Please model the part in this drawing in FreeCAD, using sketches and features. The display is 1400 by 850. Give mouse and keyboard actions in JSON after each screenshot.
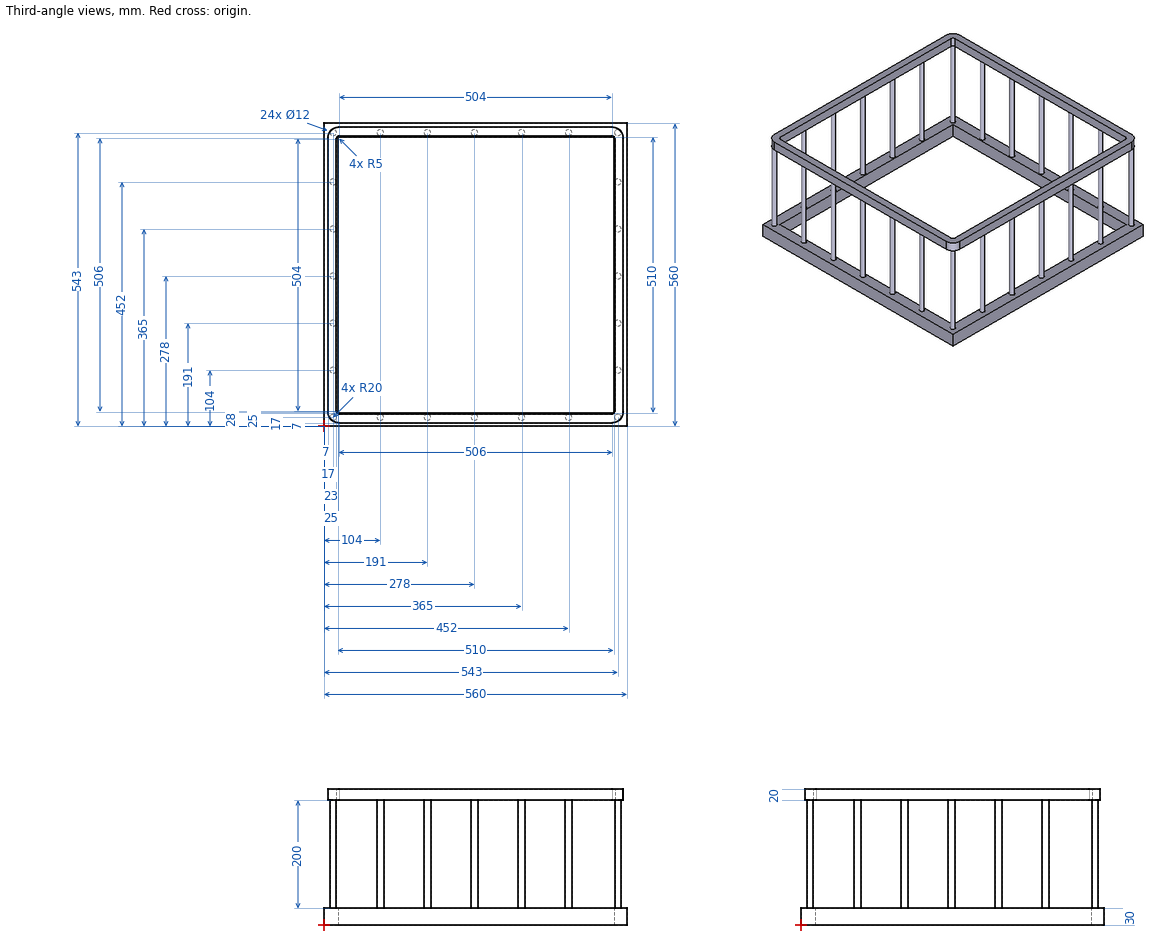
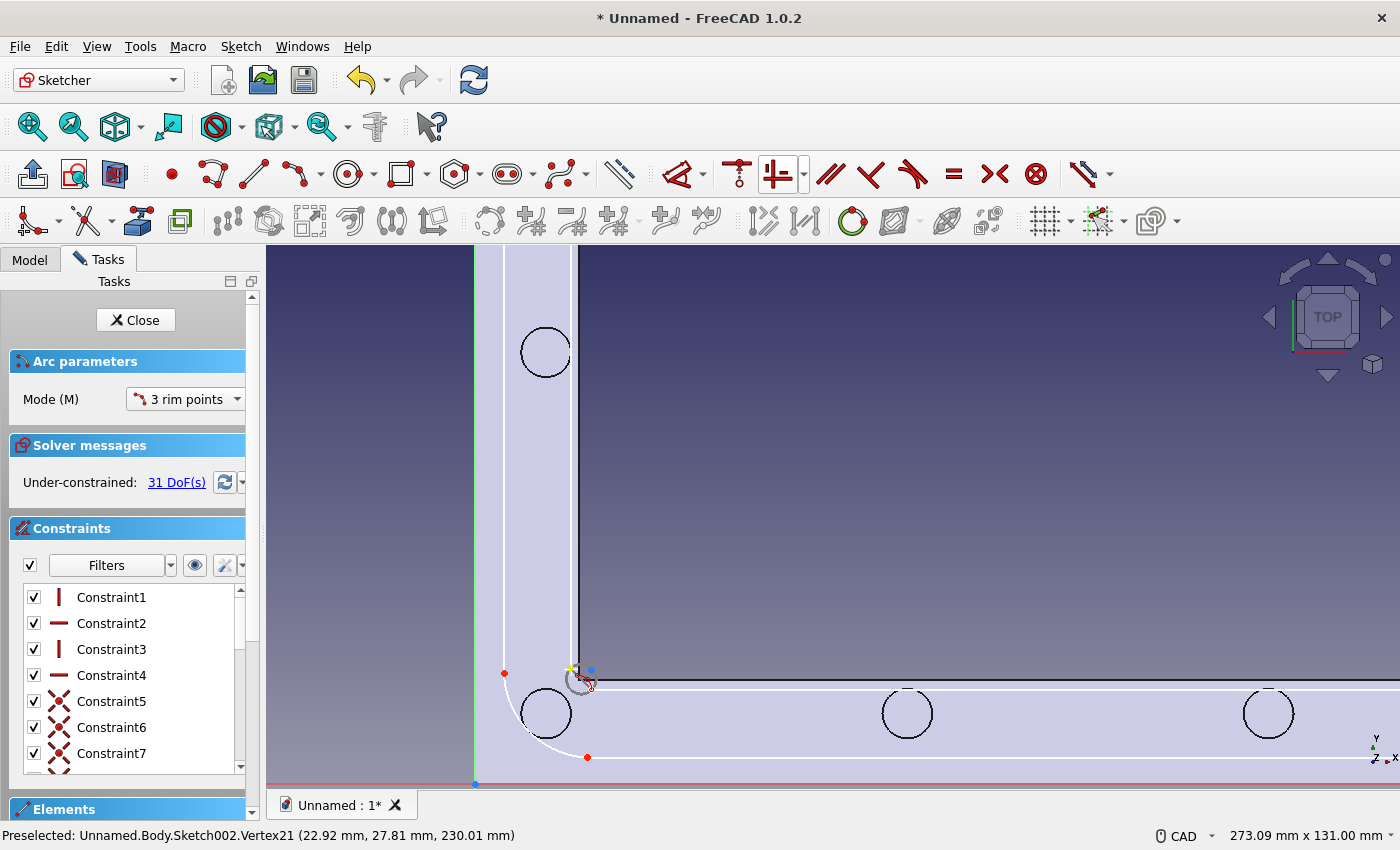
{"action": "scroll", "coordinate": [577, 683], "scroll_direction": "up", "scroll_amount": 5}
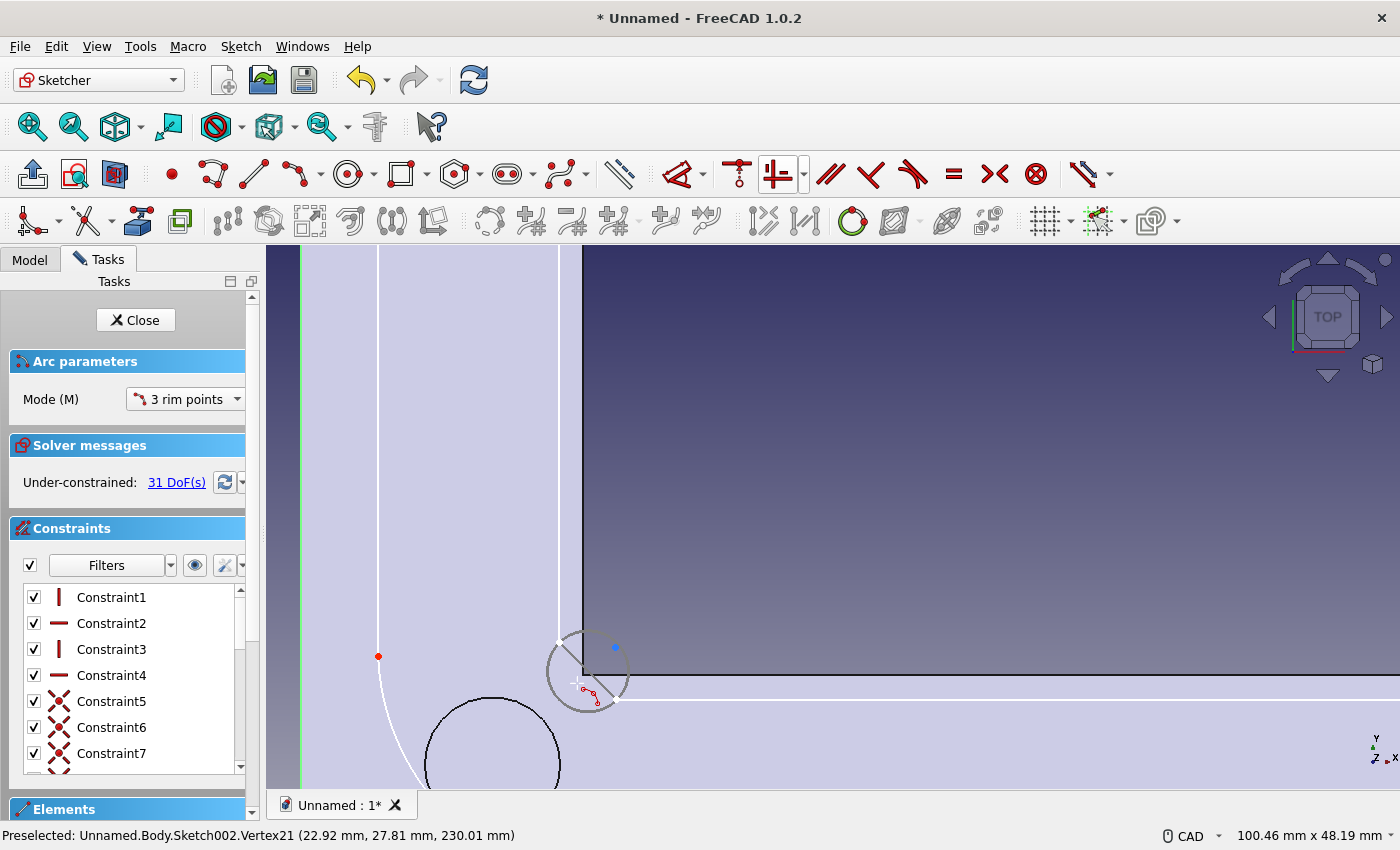
{"action": "left_click", "coordinate": [577, 681]}
{"action": "key", "text": "Escape"}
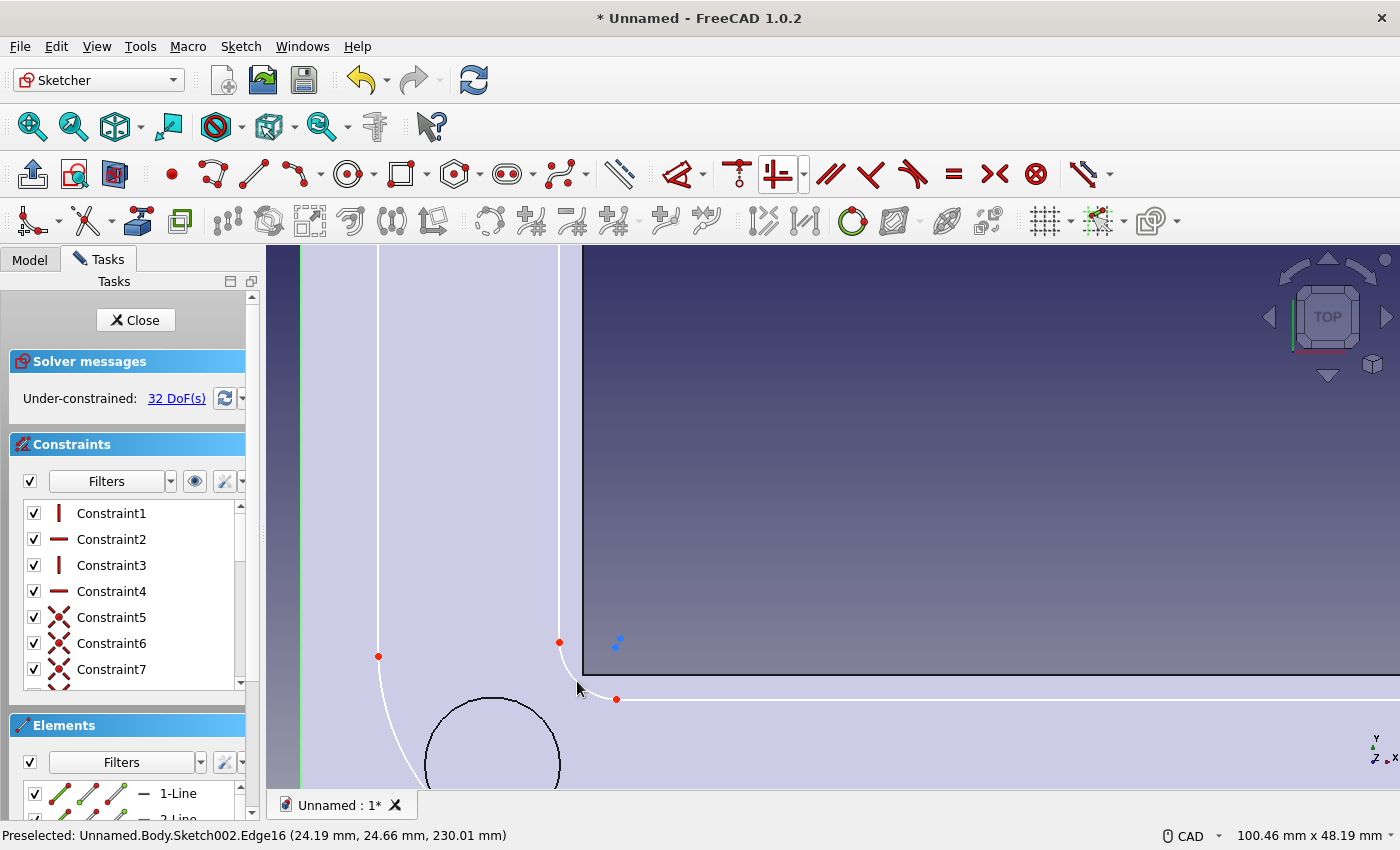
{"action": "scroll", "coordinate": [592, 691], "scroll_direction": "down", "scroll_amount": 14}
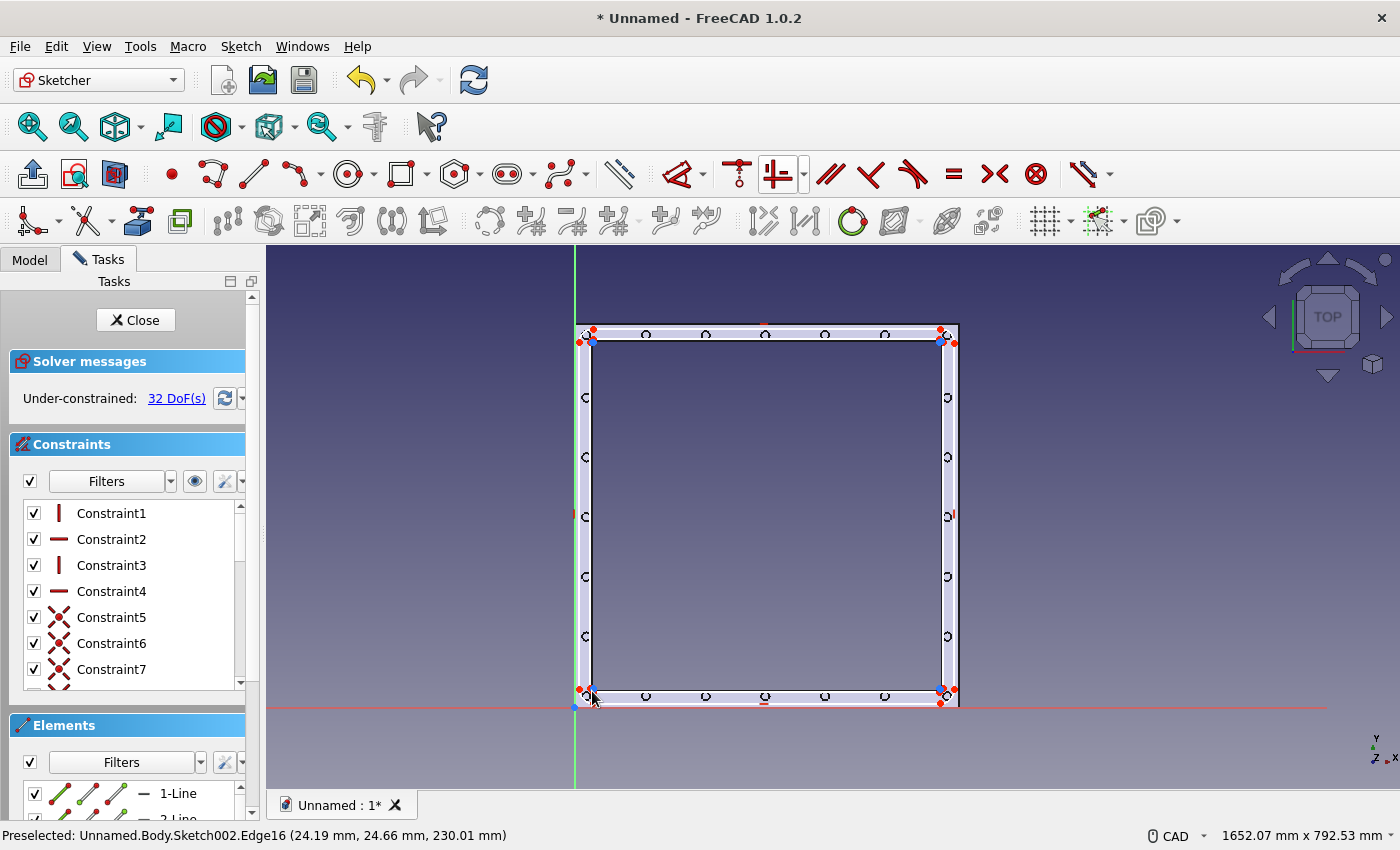
{"action": "scroll", "coordinate": [579, 447], "scroll_direction": "up", "scroll_amount": 6}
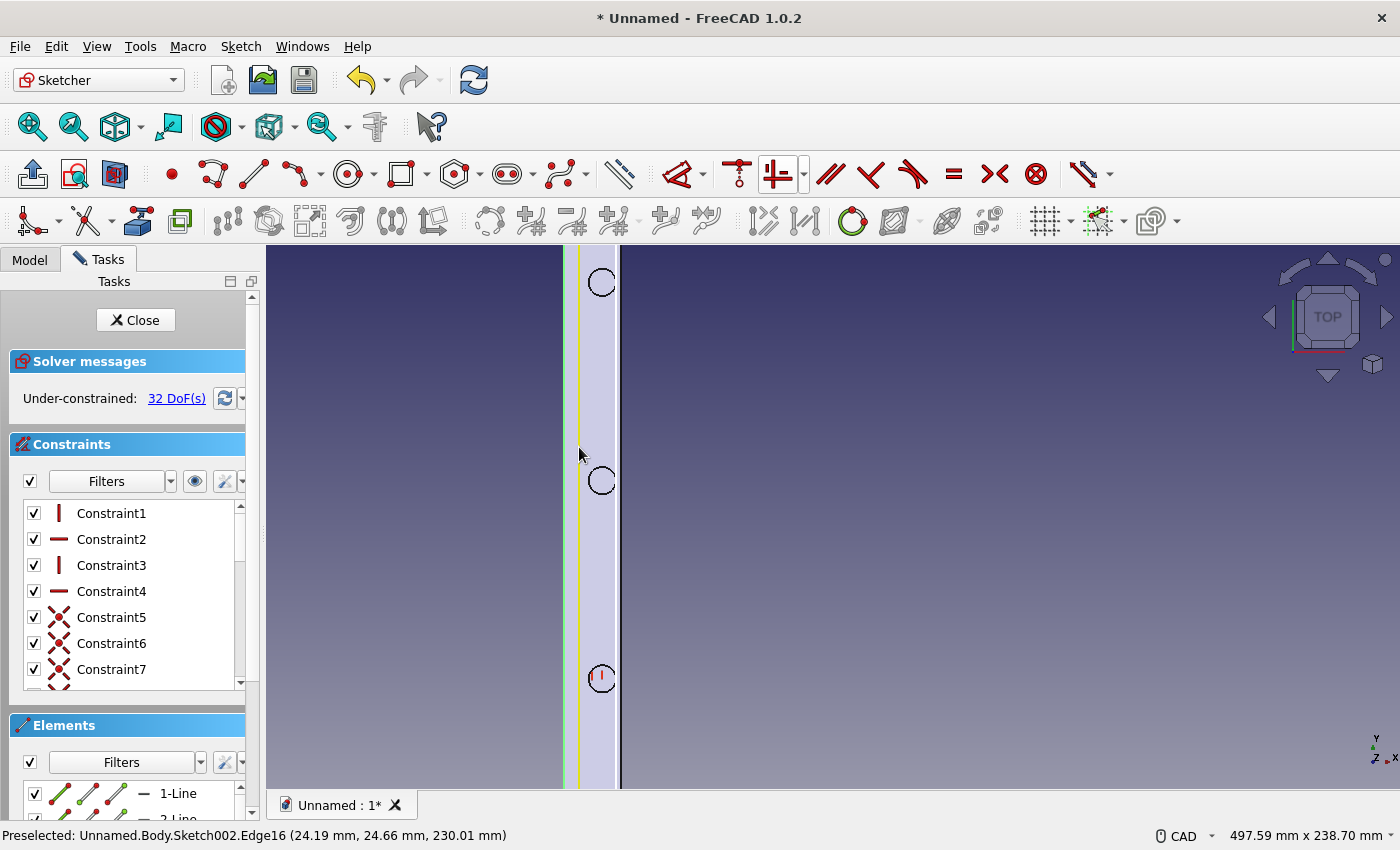
{"action": "left_click", "coordinate": [579, 445]}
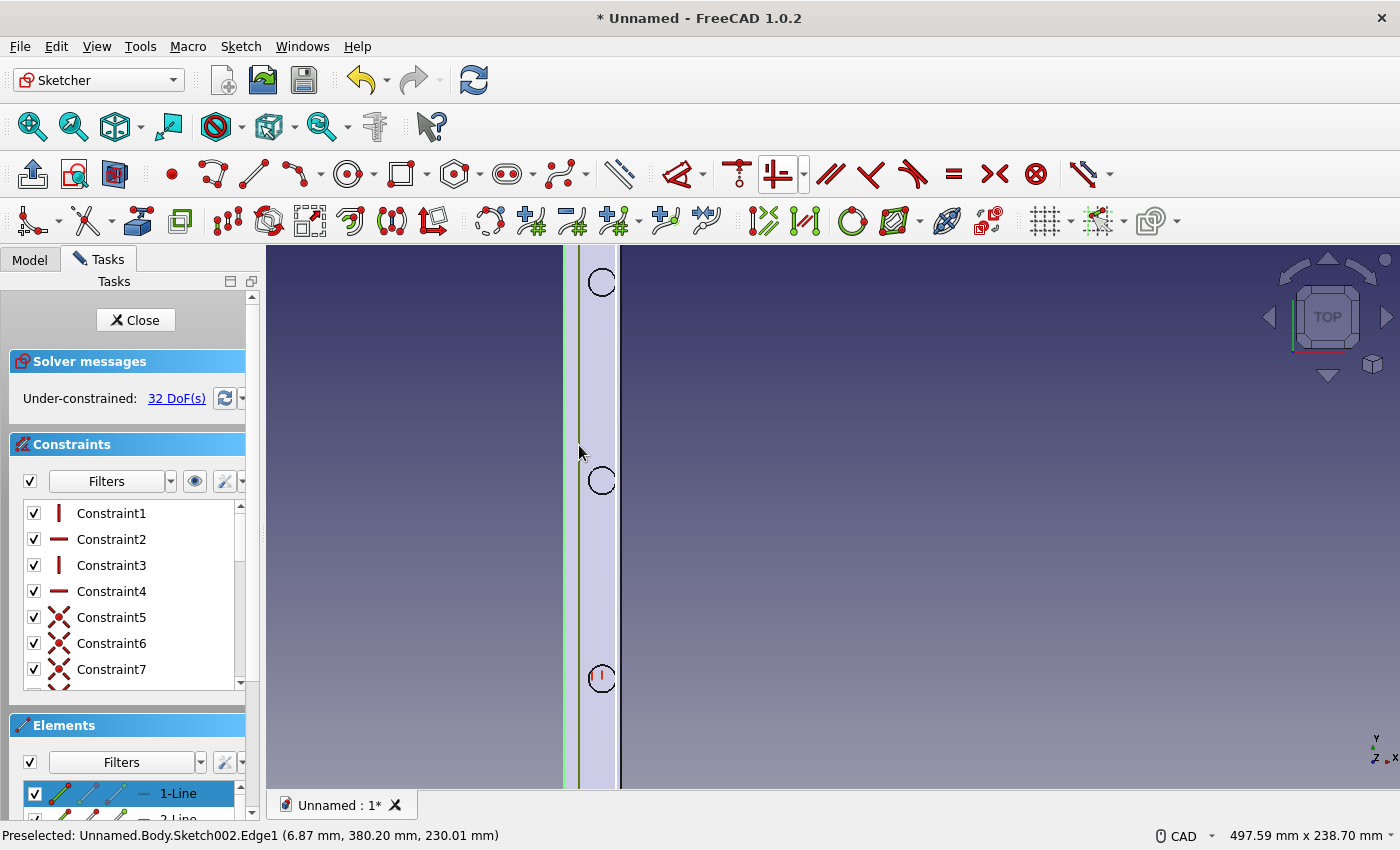
{"action": "scroll", "coordinate": [580, 446], "scroll_direction": "down", "scroll_amount": 6}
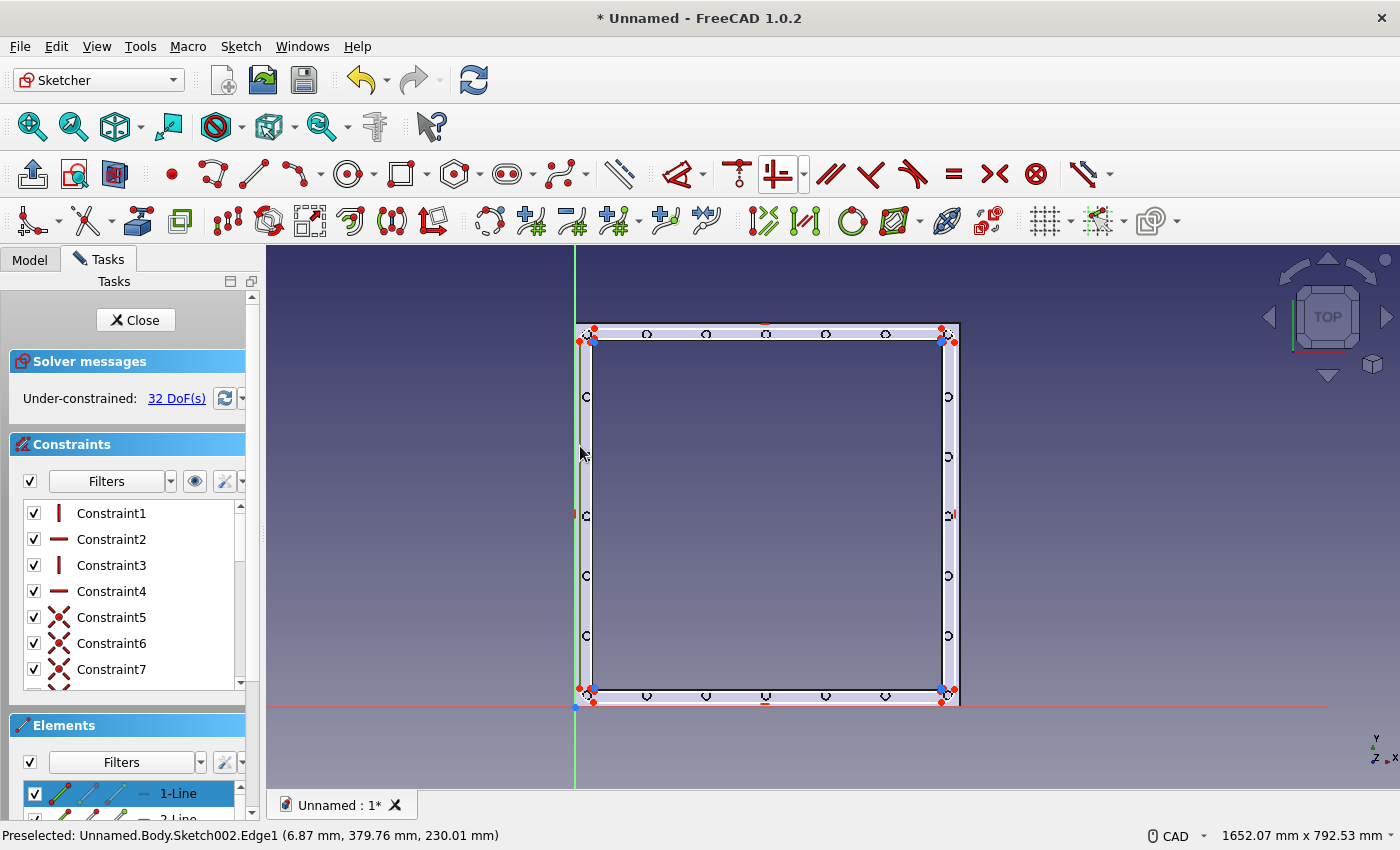
{"action": "scroll", "coordinate": [582, 695], "scroll_direction": "up", "scroll_amount": 4}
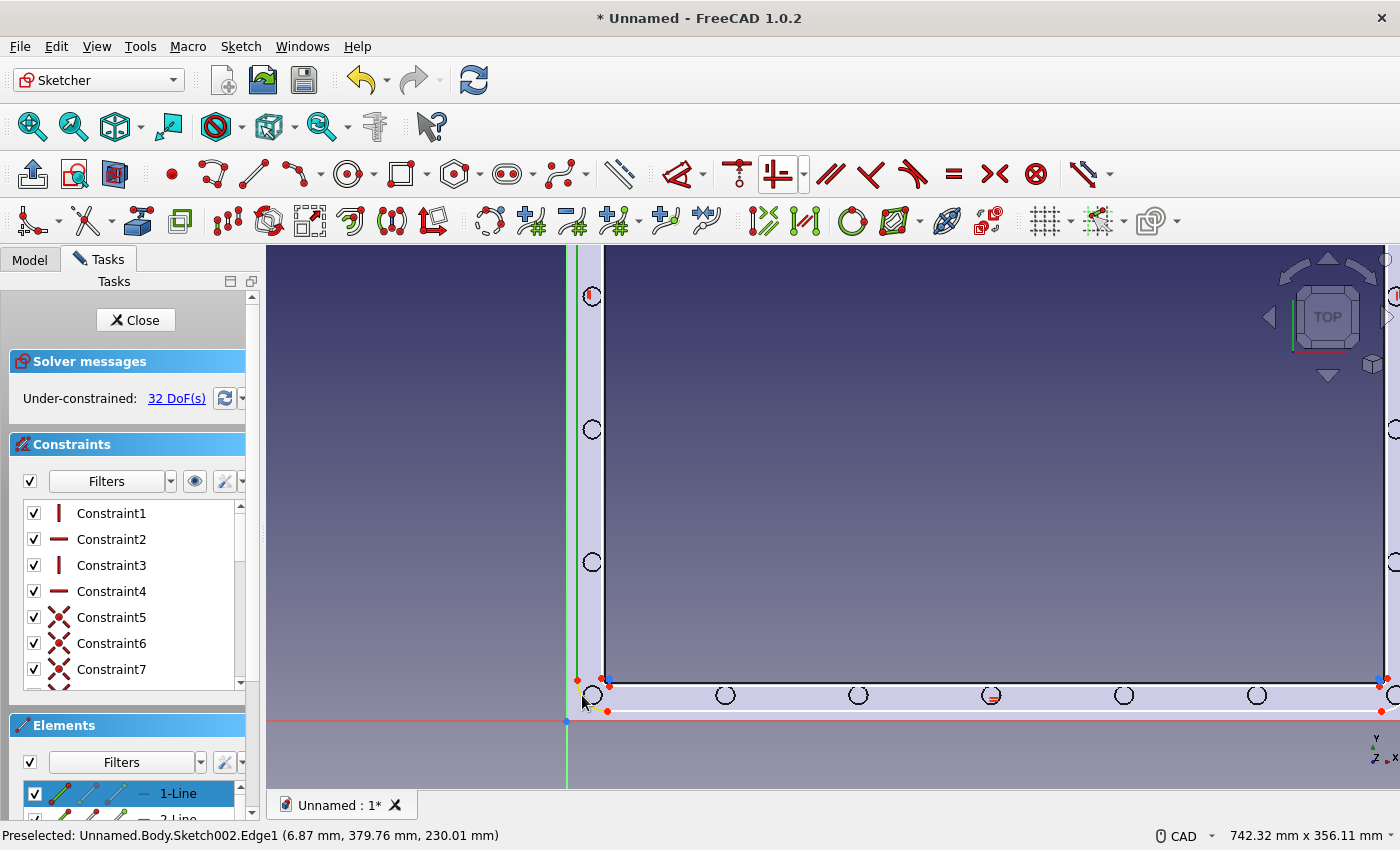
{"action": "left_click", "coordinate": [581, 694]}